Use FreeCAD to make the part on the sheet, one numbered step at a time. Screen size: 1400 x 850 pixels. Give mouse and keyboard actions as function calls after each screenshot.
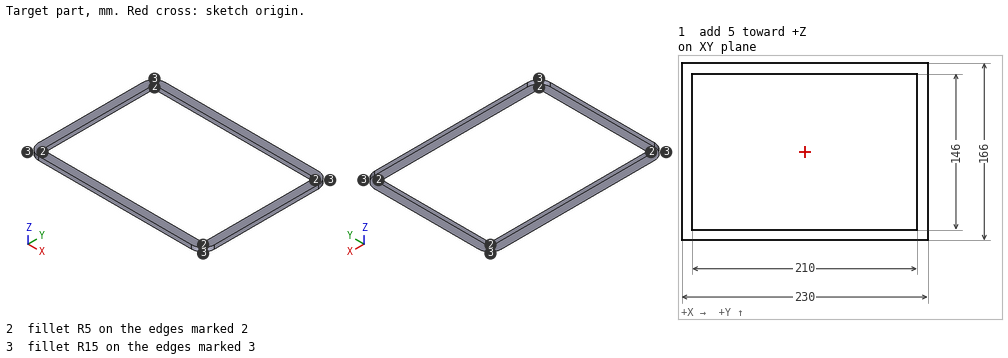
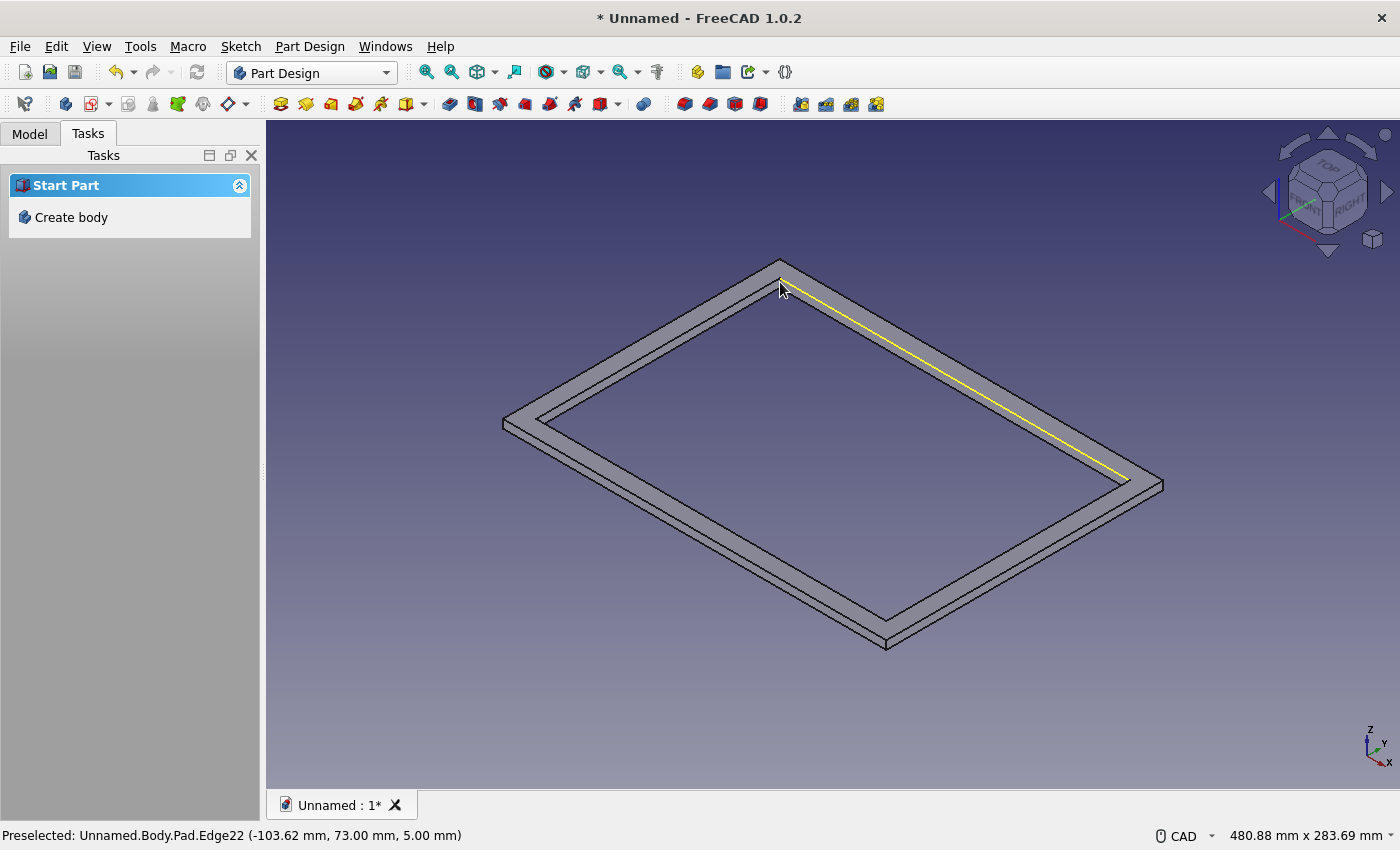
key(2)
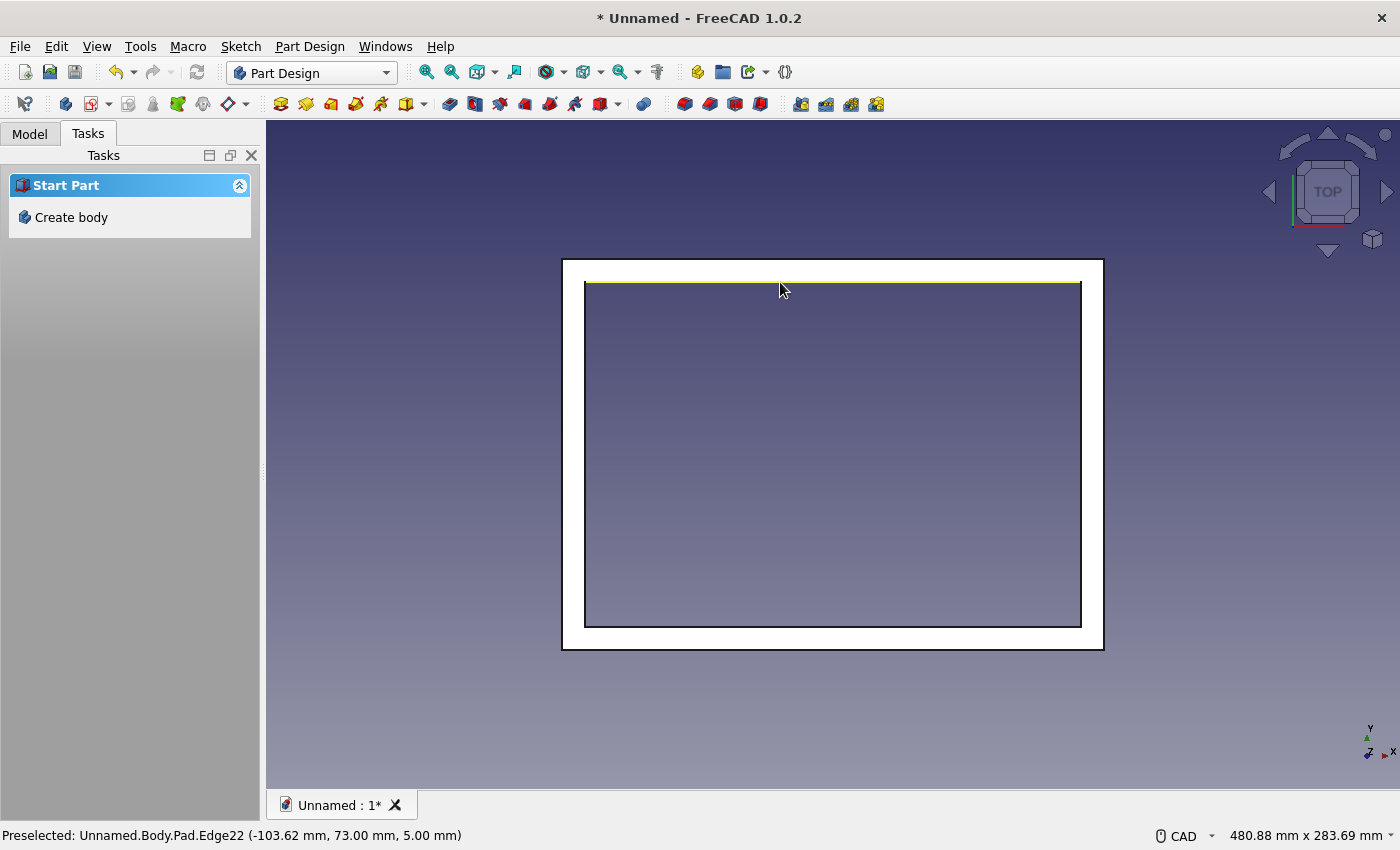
scroll(585, 281, up, 7)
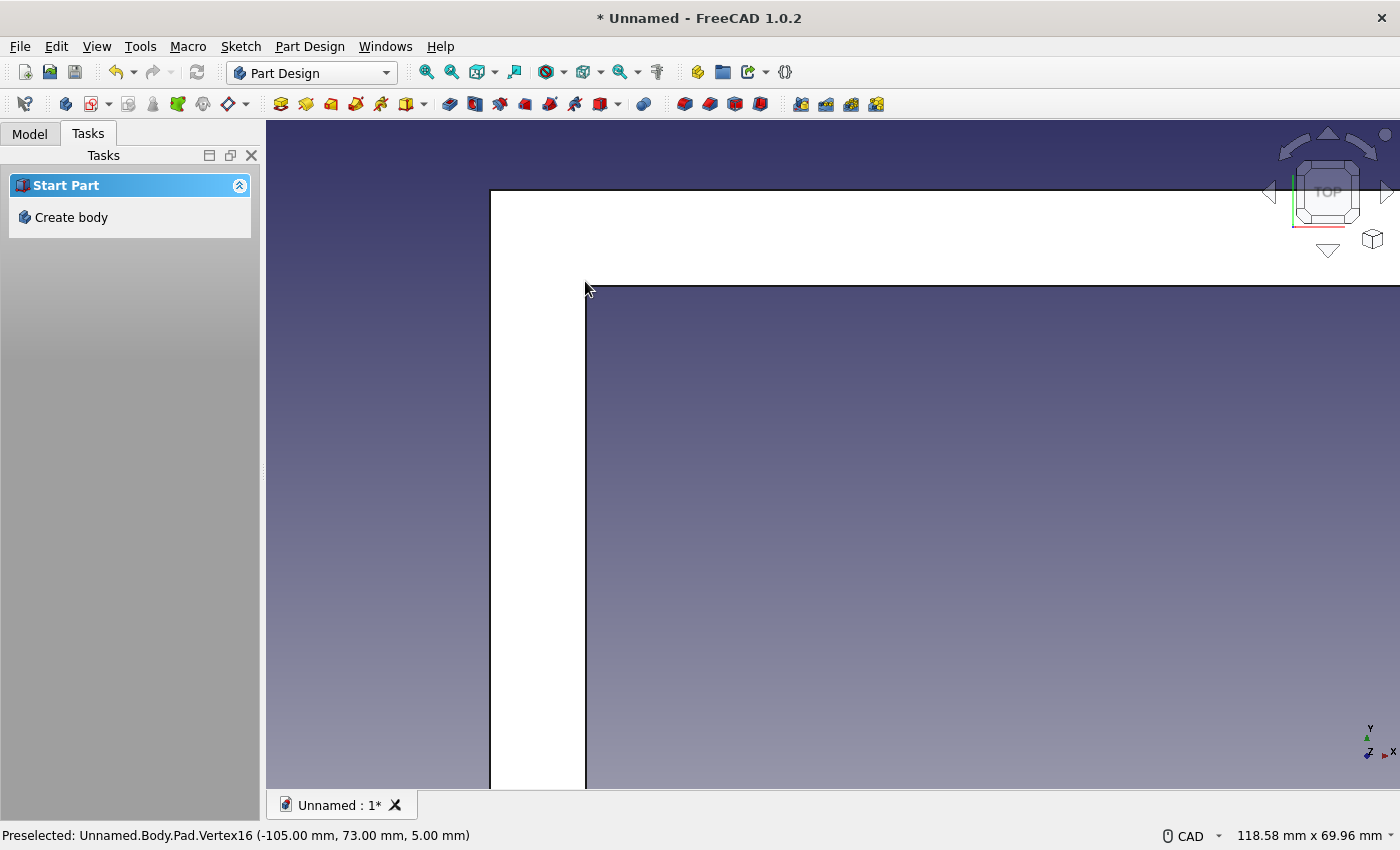
key(v)
key(f)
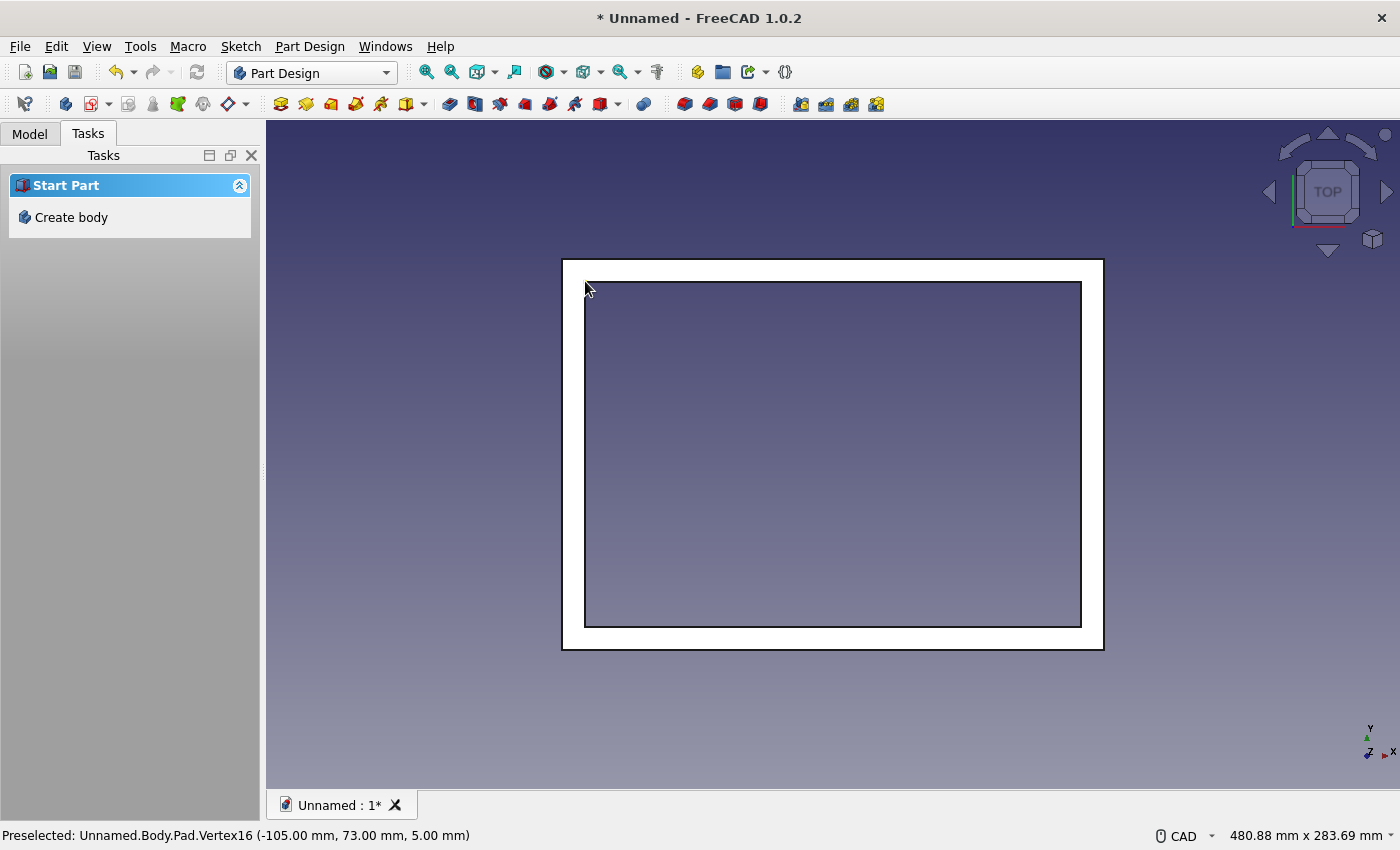
key(1)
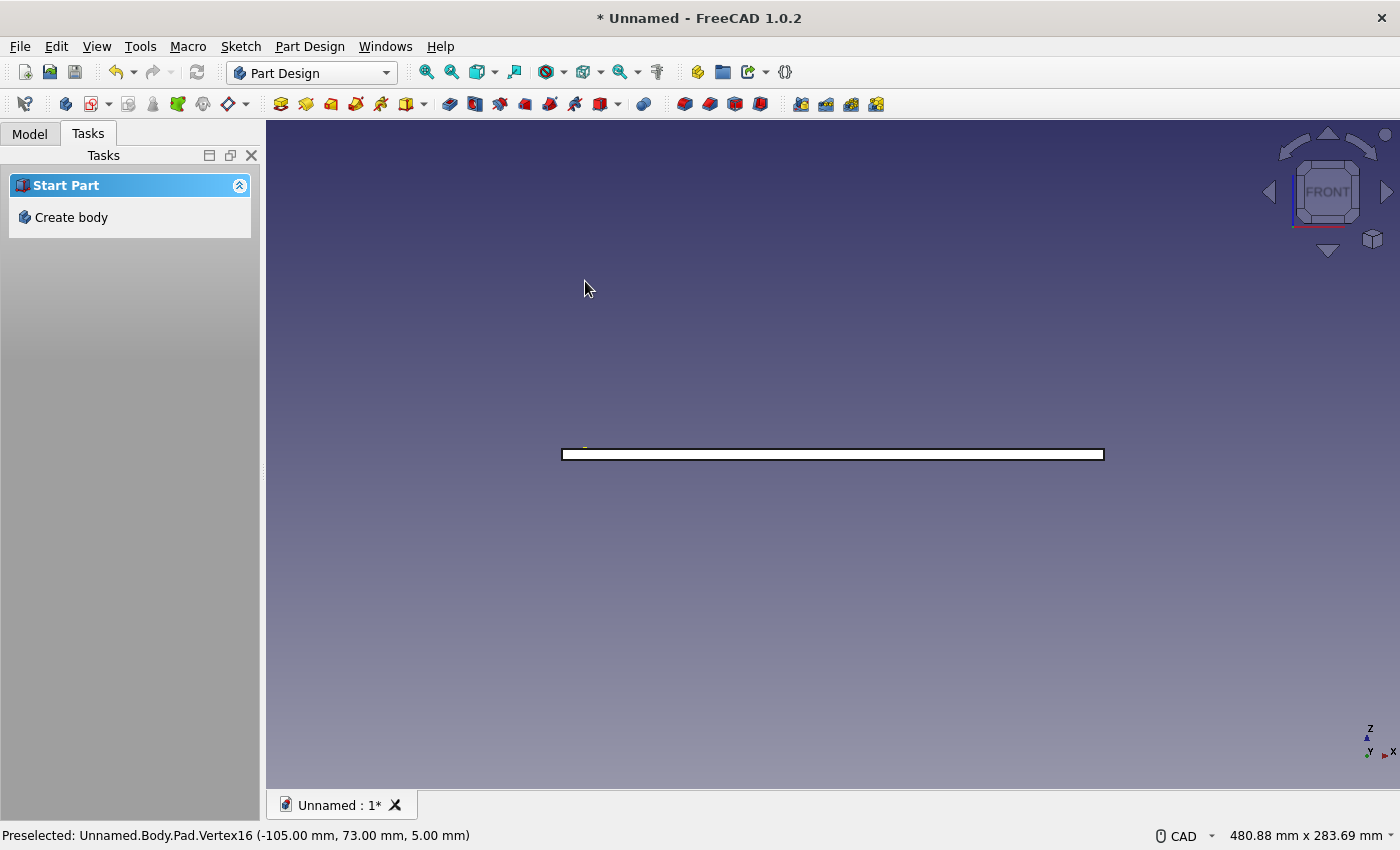
scroll(585, 453, up, 7)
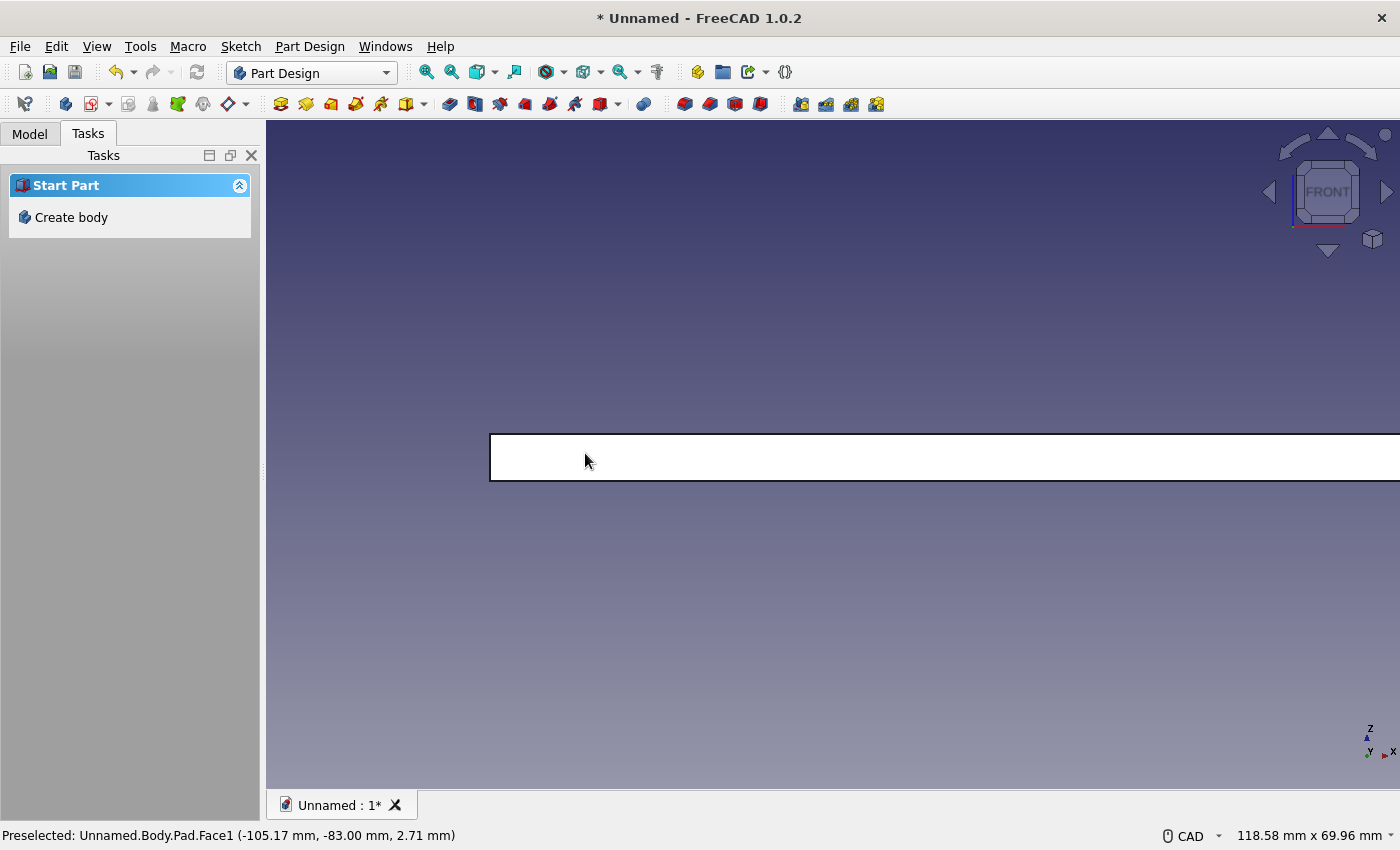
key(v)
key(f)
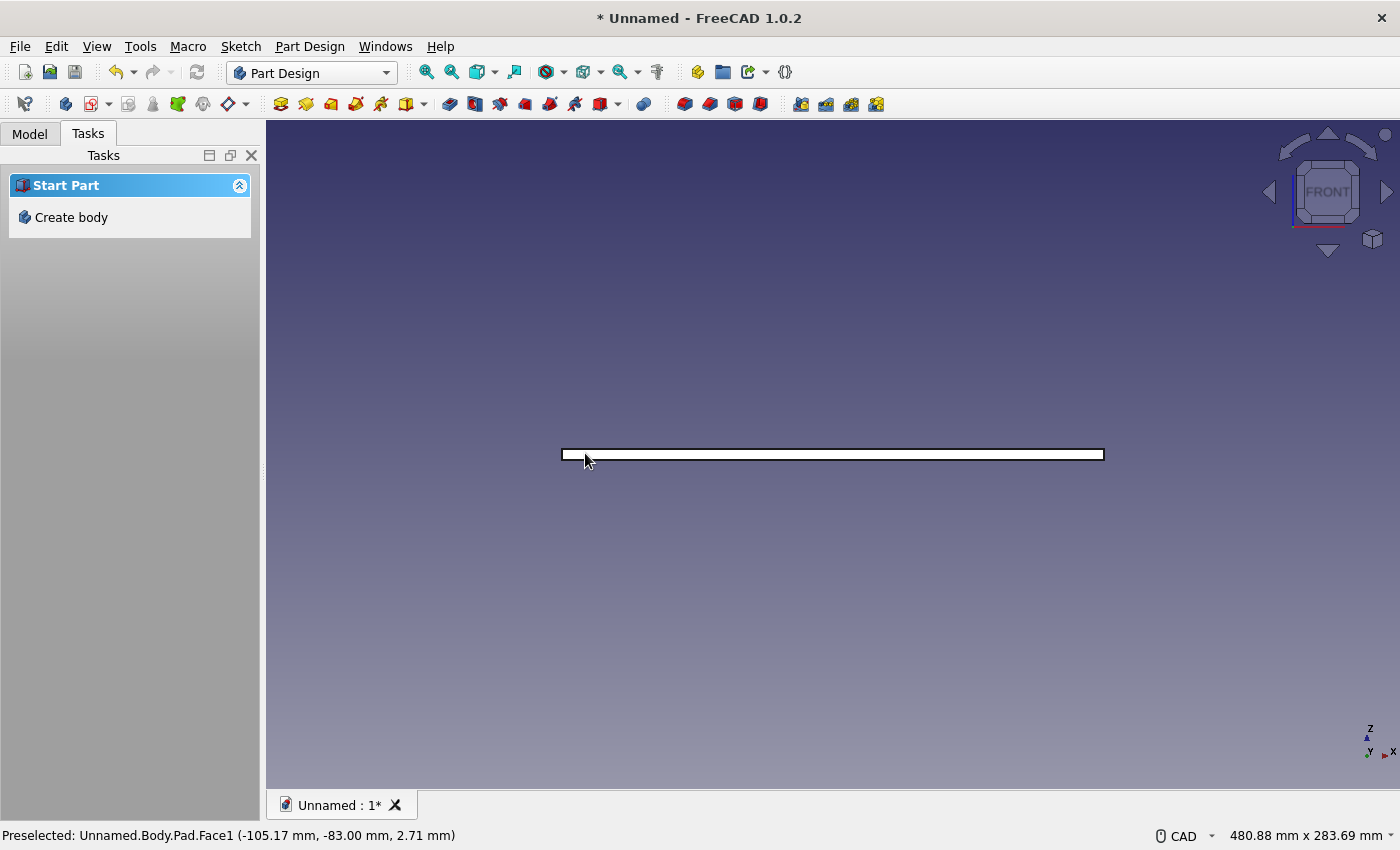
key(3)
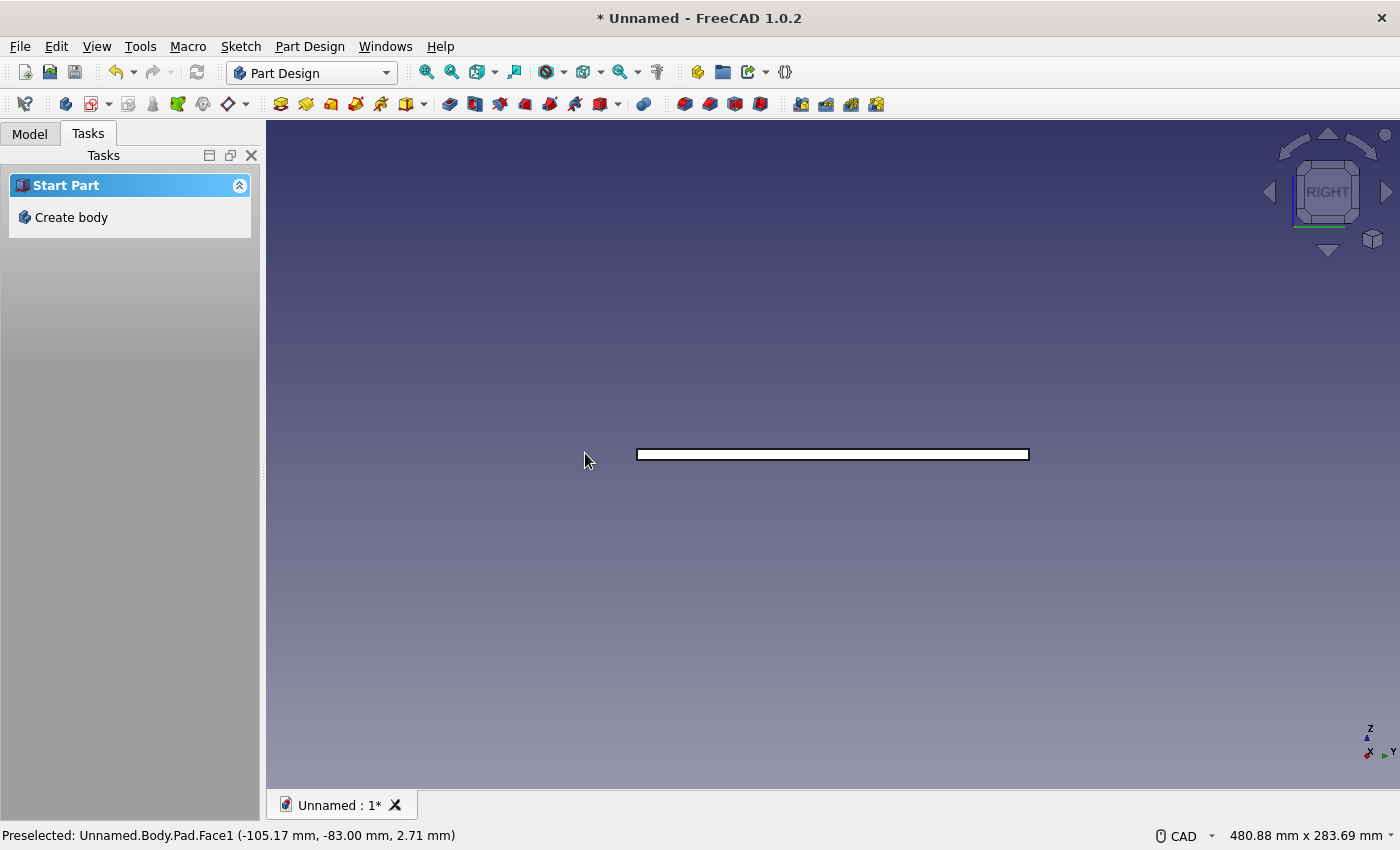
key(v)
key(f)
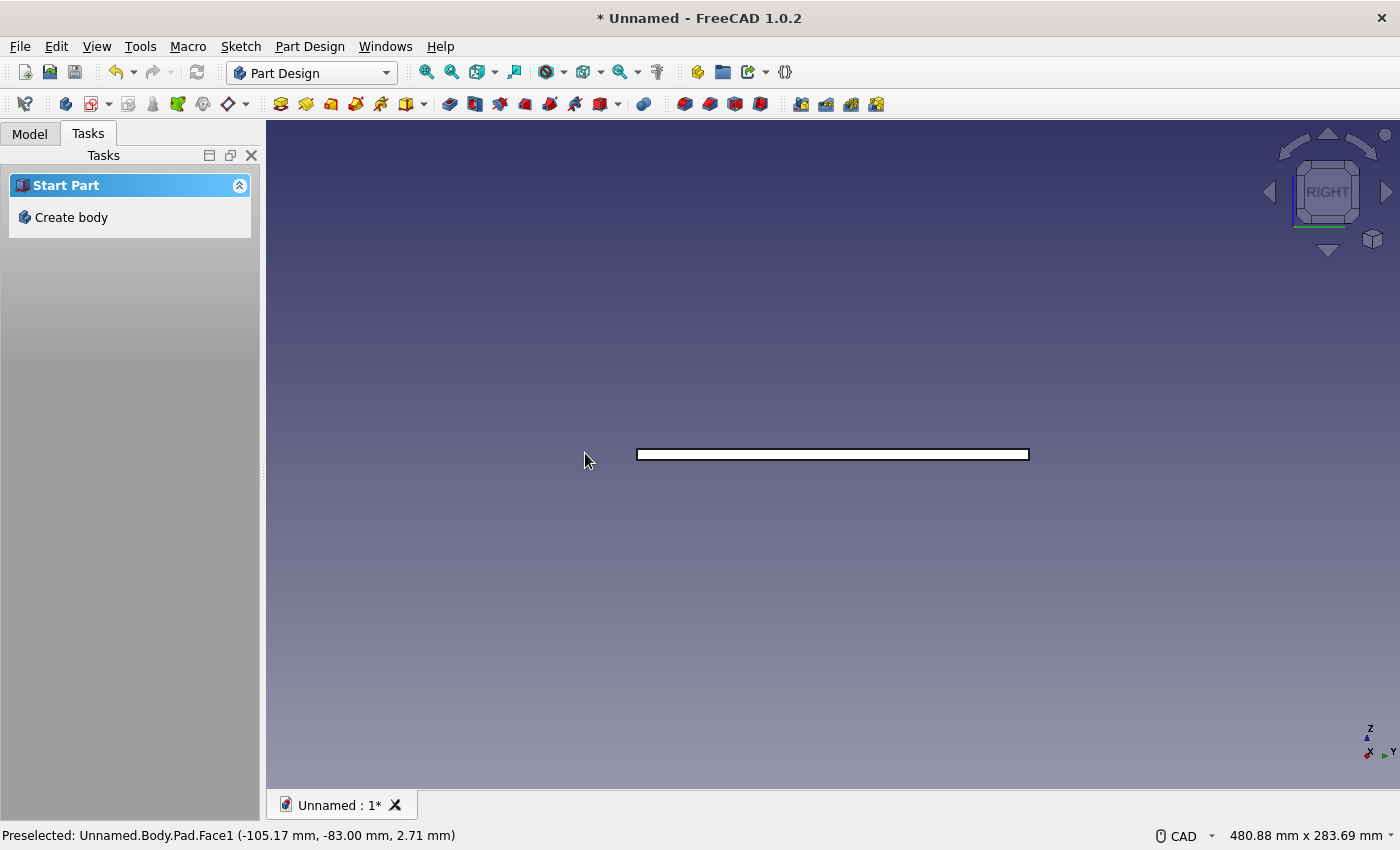
scroll(1005, 453, up, 7)